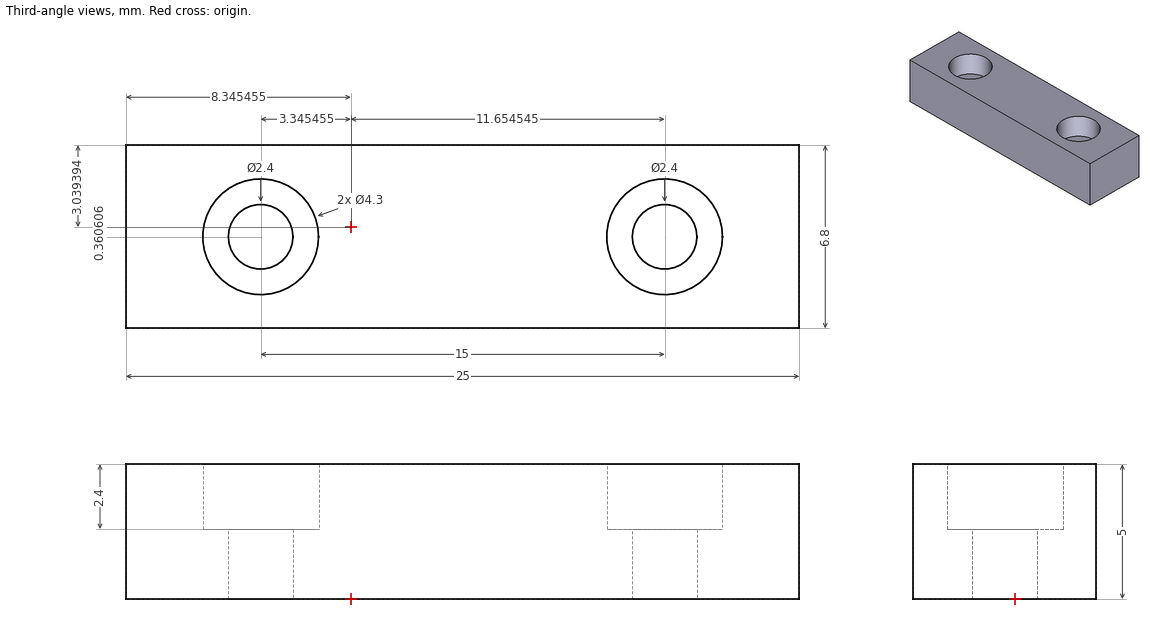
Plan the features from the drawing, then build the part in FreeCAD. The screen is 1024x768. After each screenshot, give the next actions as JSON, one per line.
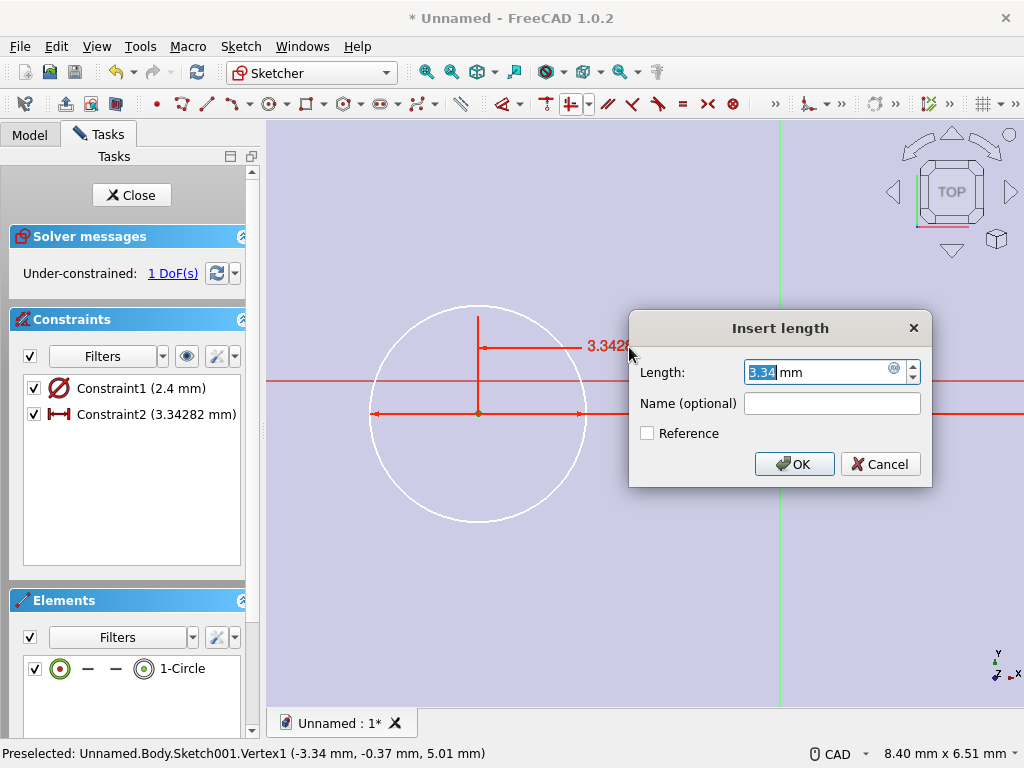
{"action": "type", "text": "3.345455"}
{"action": "key", "text": "Return"}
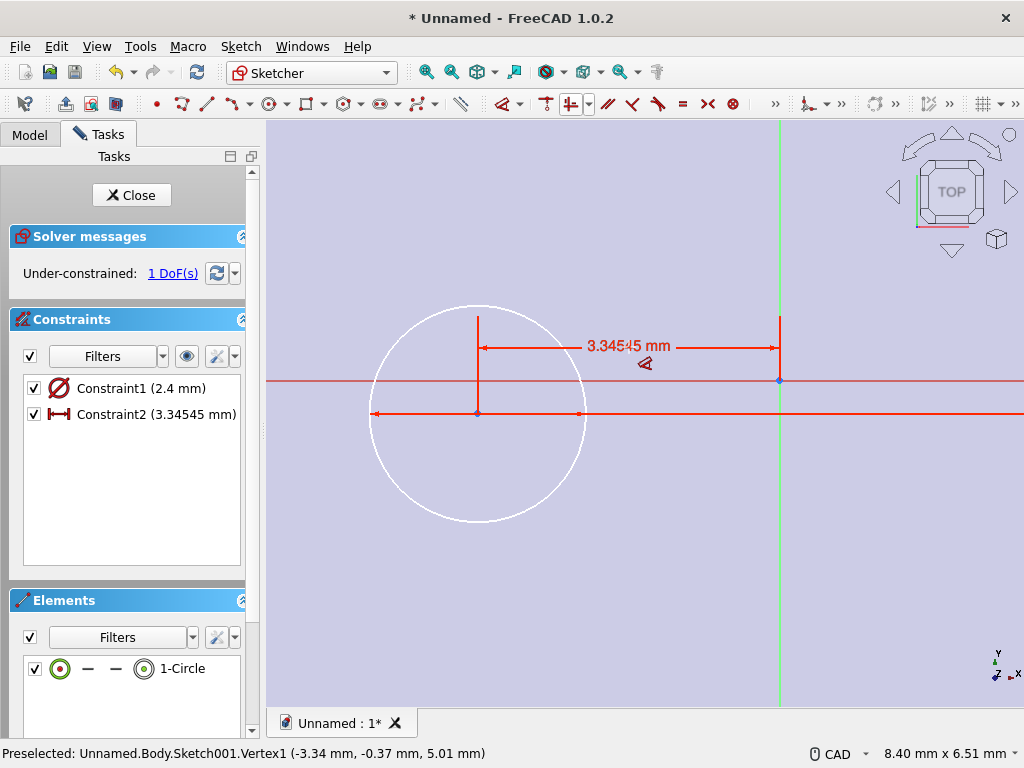
{"action": "left_click", "coordinate": [478, 414]}
{"action": "left_click", "coordinate": [814, 397]}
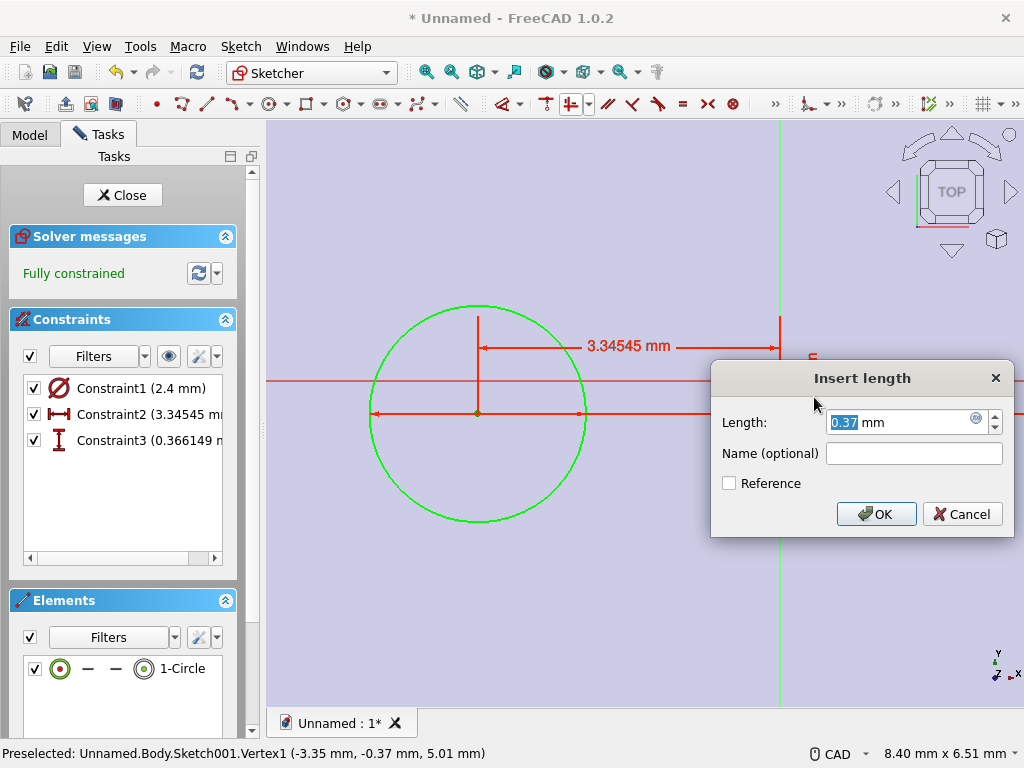
{"action": "type", "text": "0.360606"}
{"action": "key", "text": "Return"}
{"action": "key", "text": "Escape"}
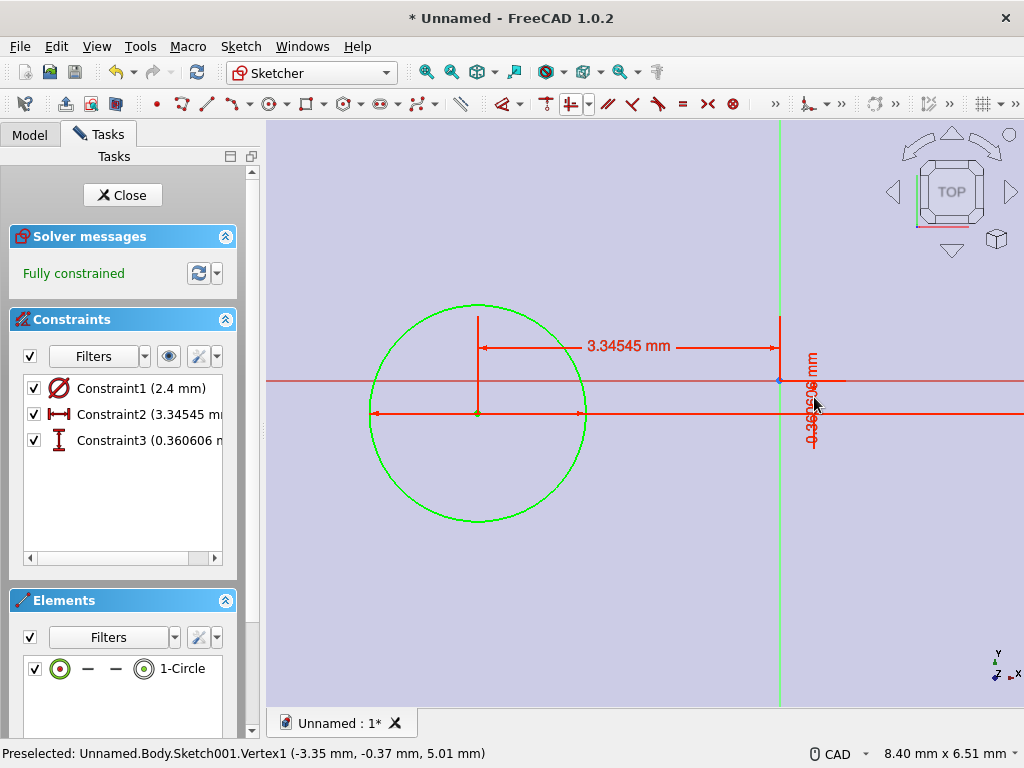
{"action": "left_click", "coordinate": [123, 195]}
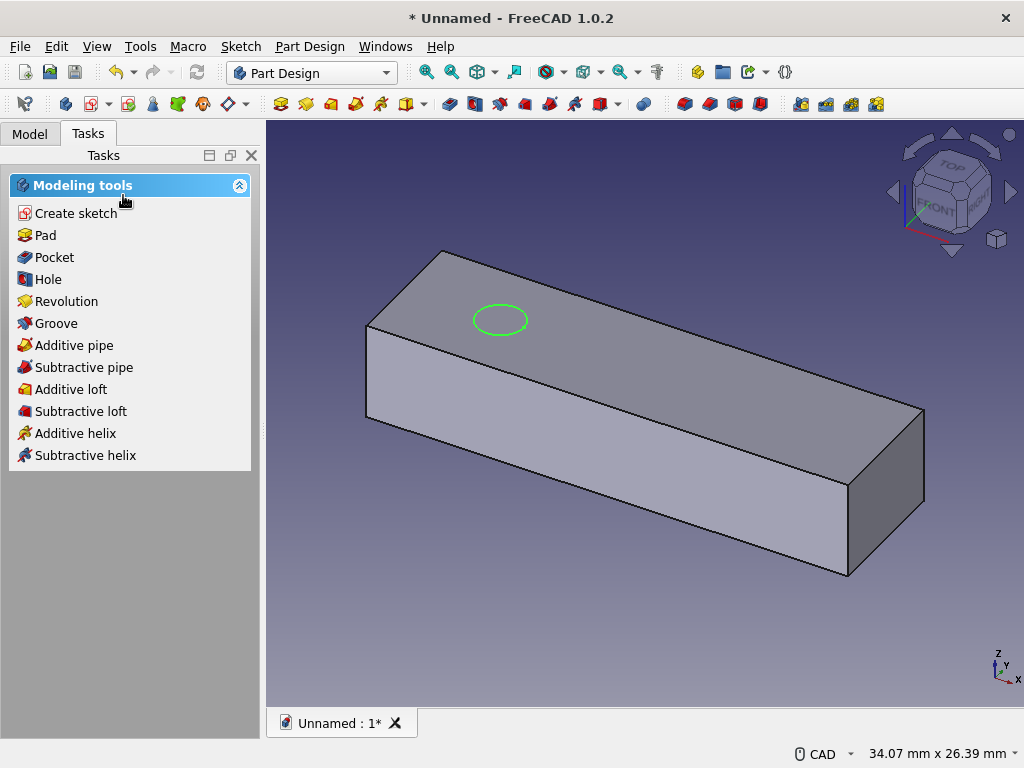
{"action": "left_click", "coordinate": [450, 104]}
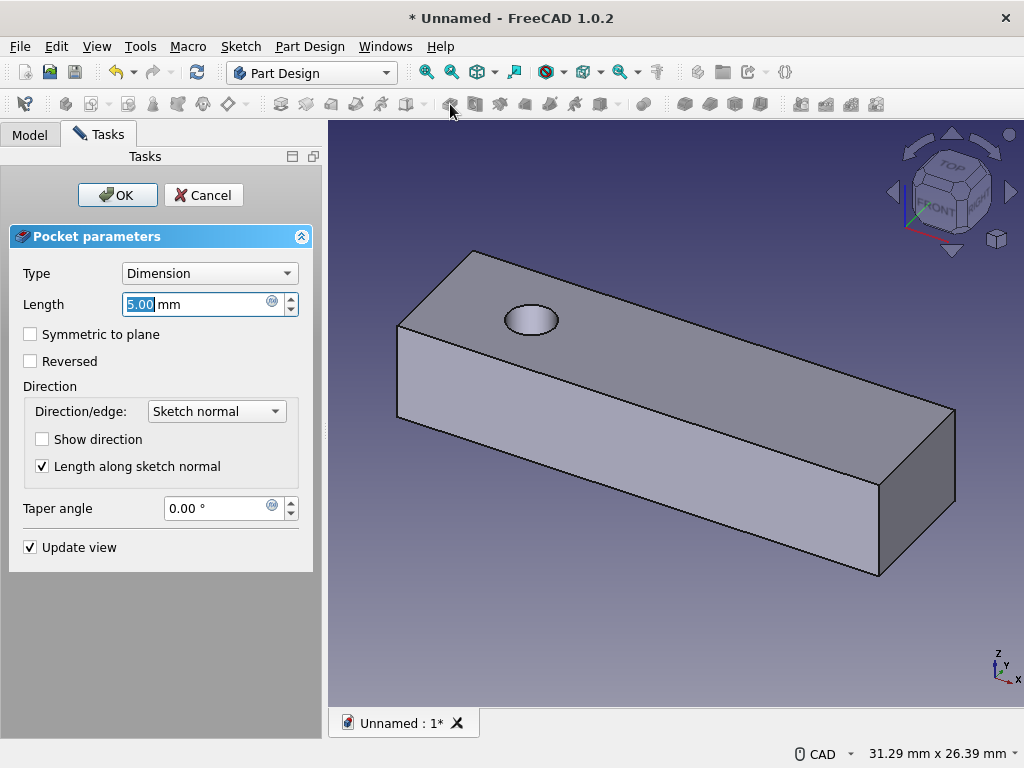
{"action": "left_click", "coordinate": [210, 274]}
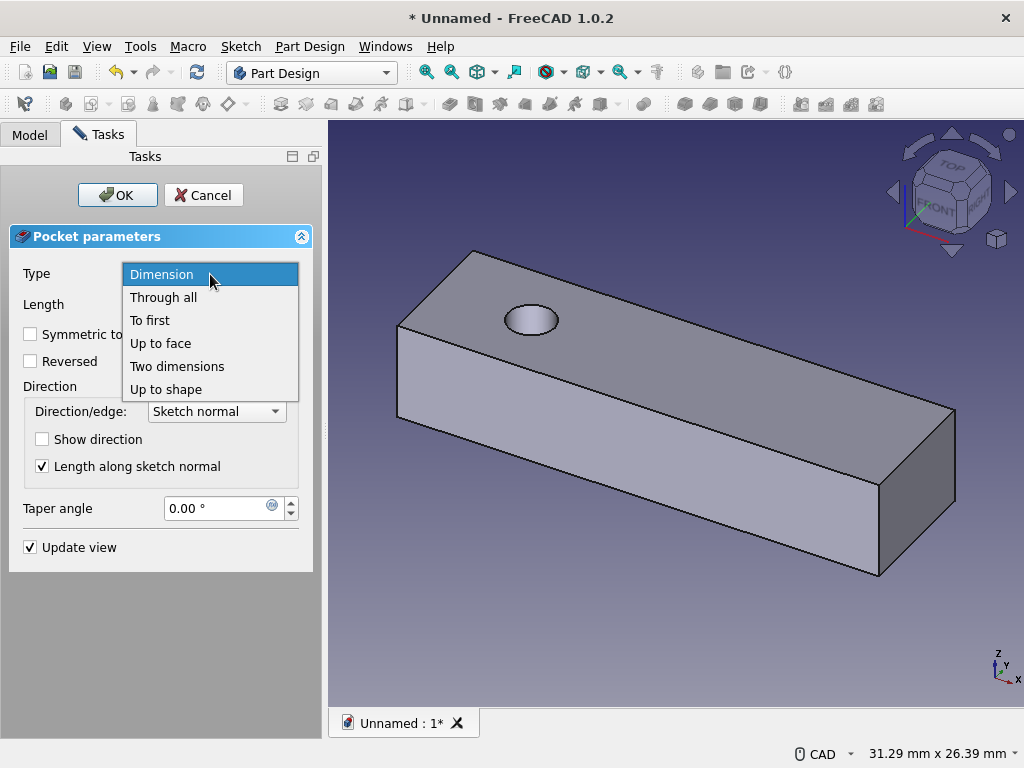
{"action": "left_click", "coordinate": [208, 320]}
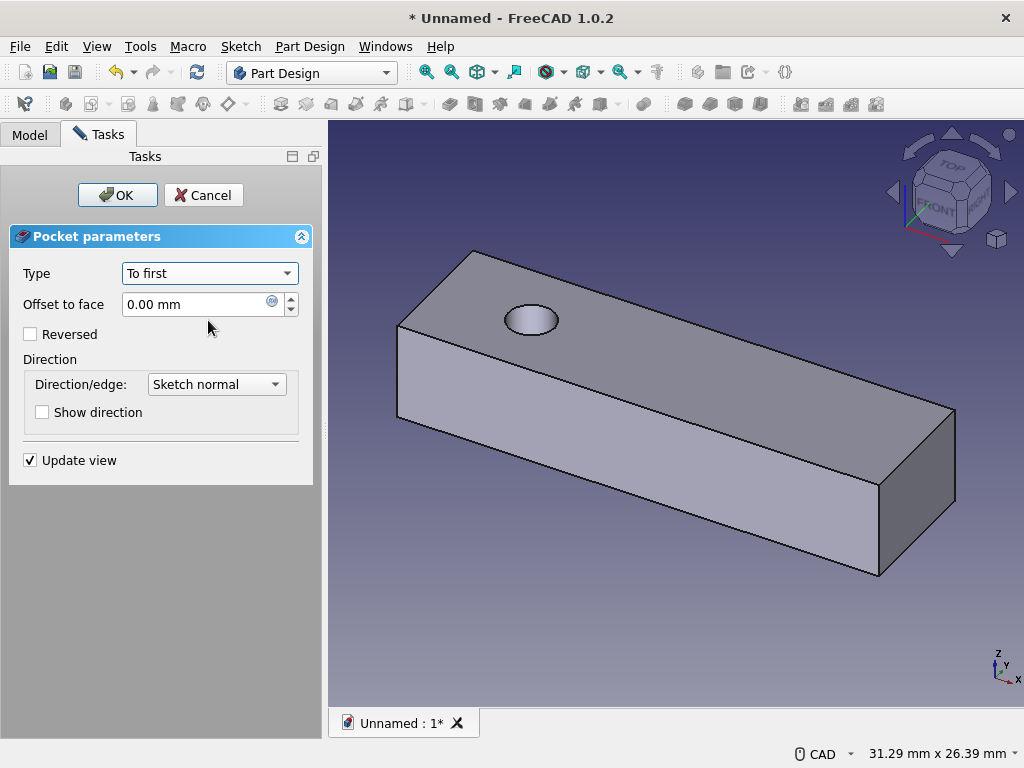
{"action": "left_click", "coordinate": [118, 195]}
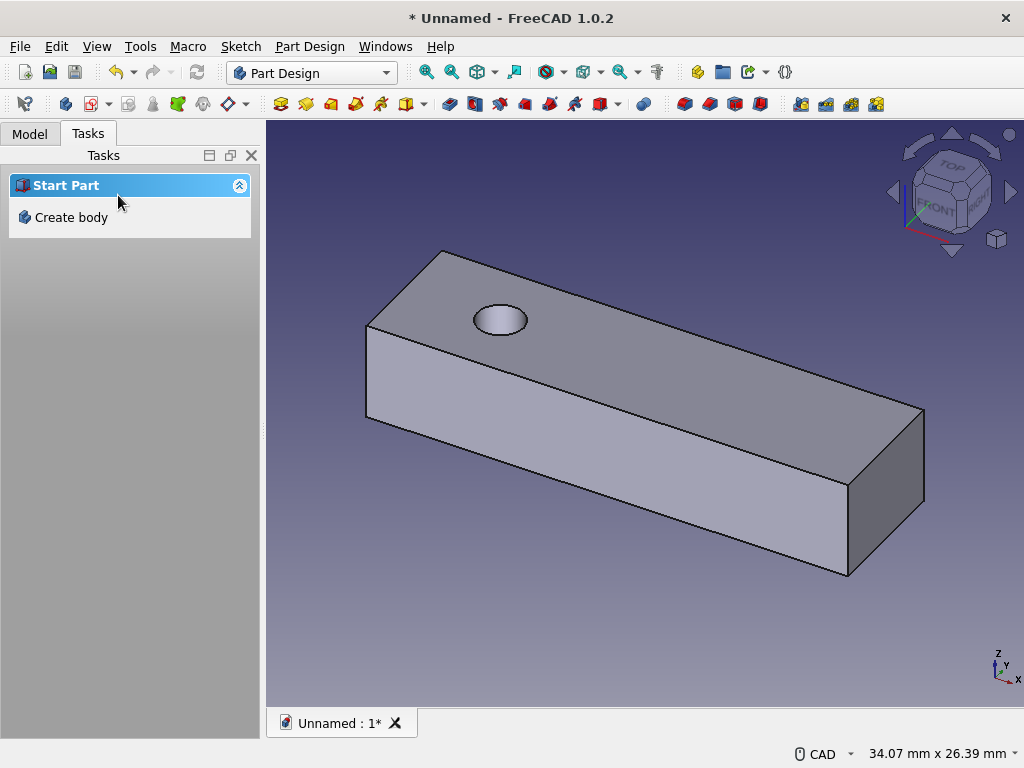
{"action": "left_click", "coordinate": [783, 413]}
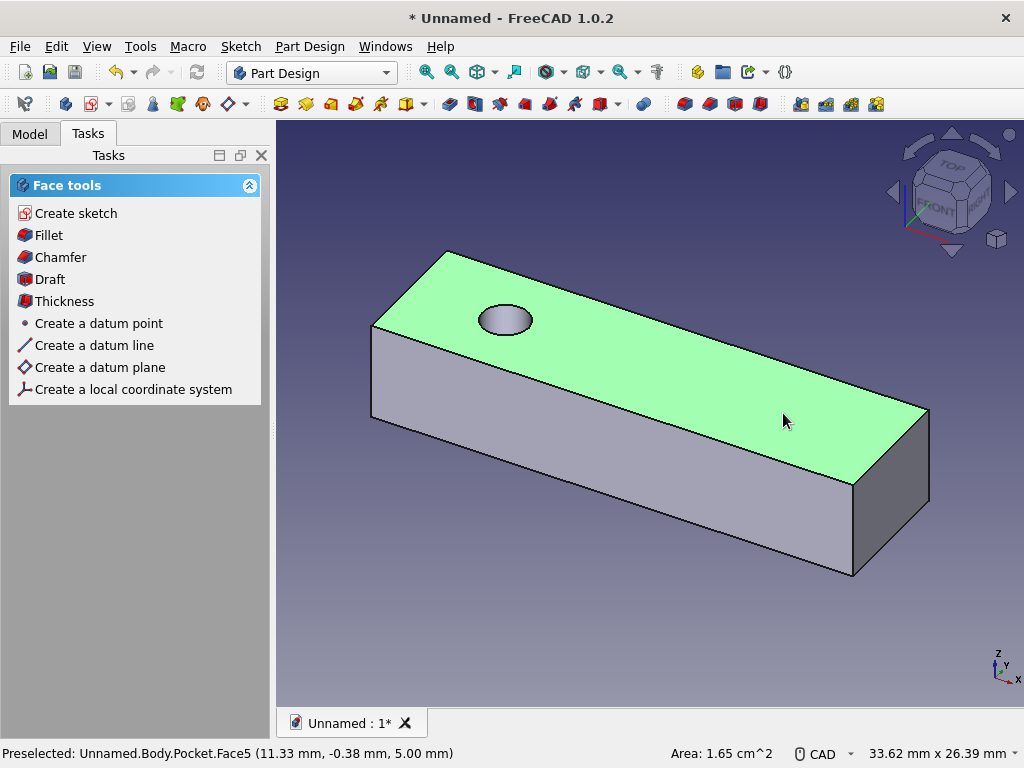
{"action": "left_click", "coordinate": [90, 104]}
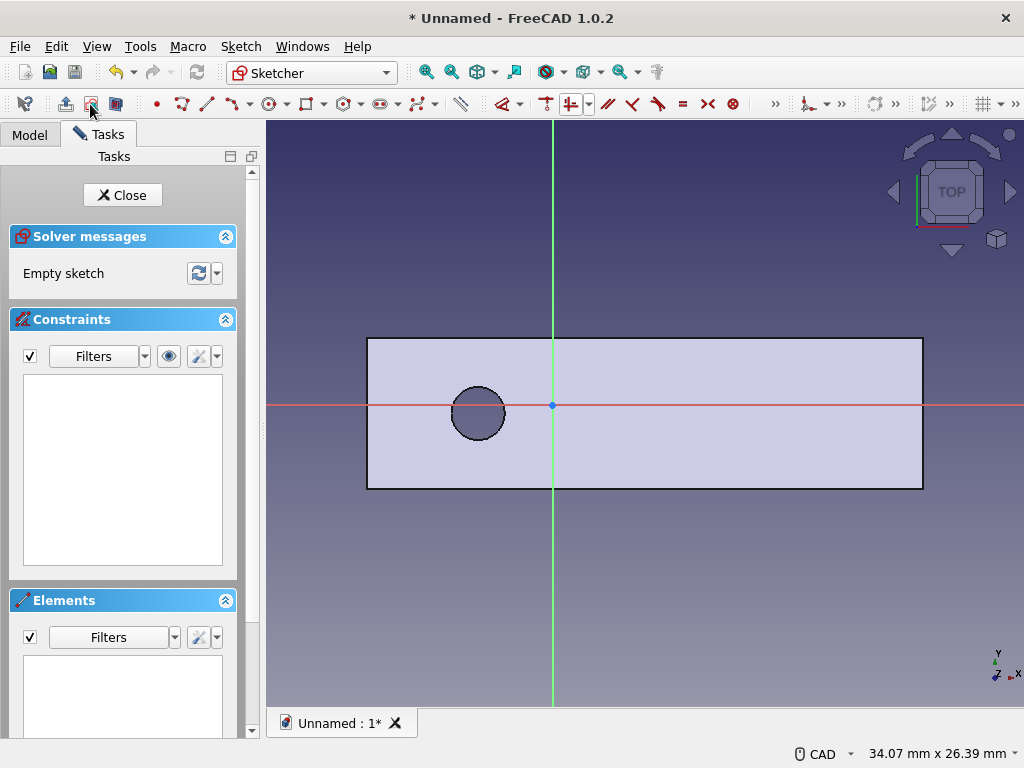
{"action": "scroll", "coordinate": [849, 413], "scroll_direction": "up", "scroll_amount": 10}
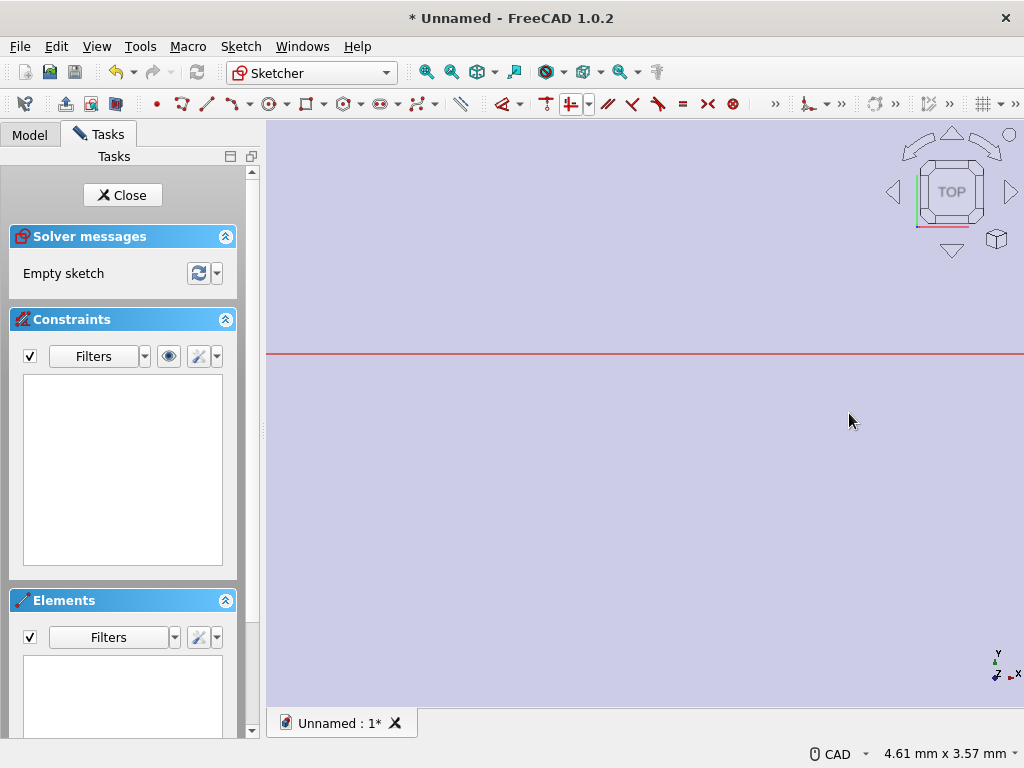
{"action": "left_click", "coordinate": [268, 104]}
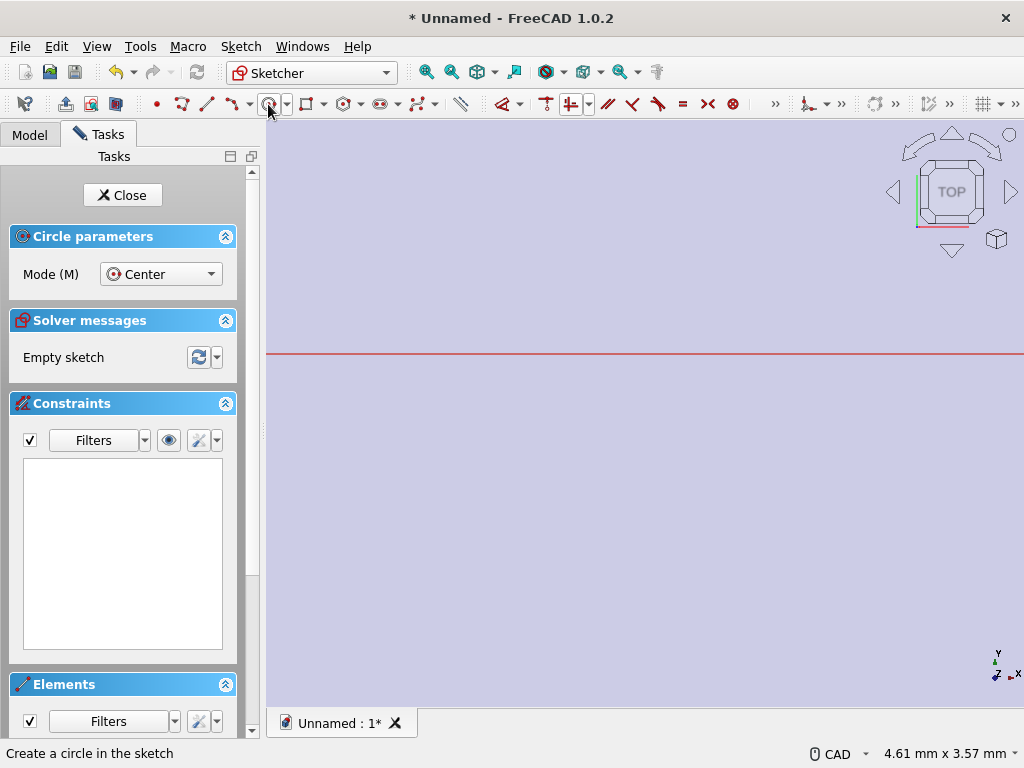
{"action": "left_click", "coordinate": [570, 413]}
{"action": "mouse_move", "coordinate": [709, 274]}